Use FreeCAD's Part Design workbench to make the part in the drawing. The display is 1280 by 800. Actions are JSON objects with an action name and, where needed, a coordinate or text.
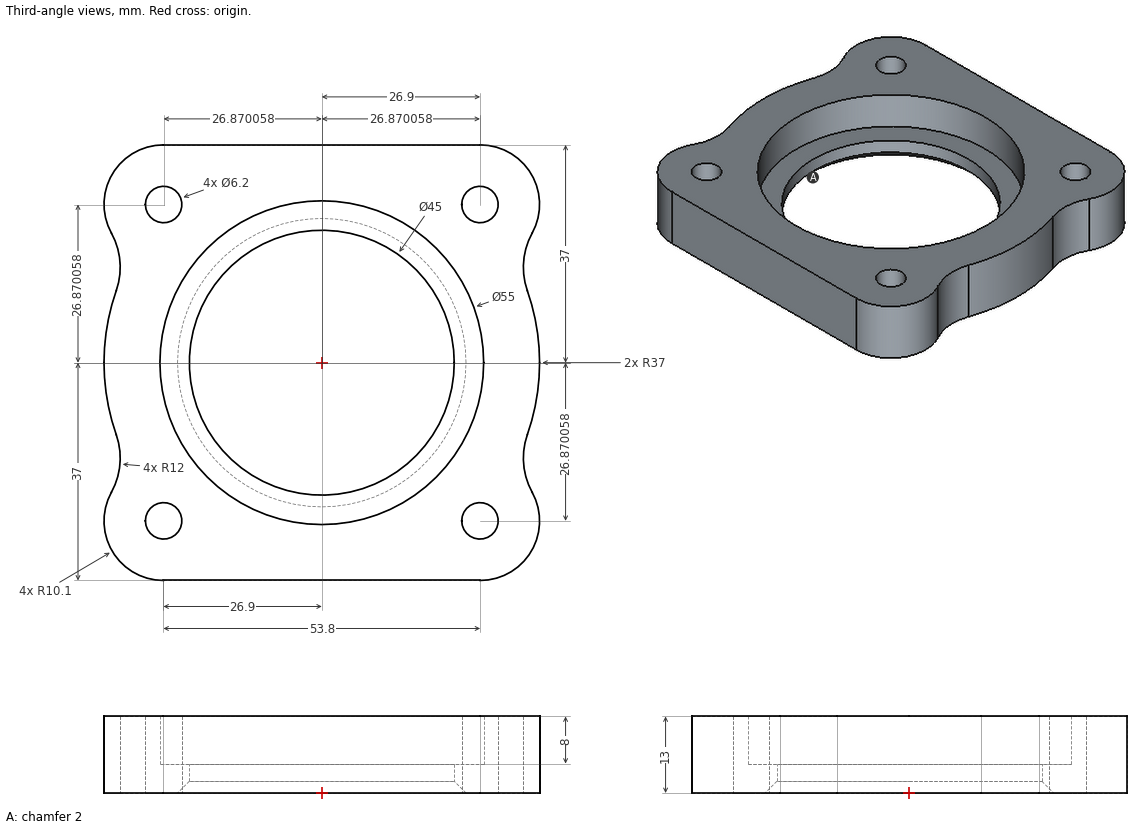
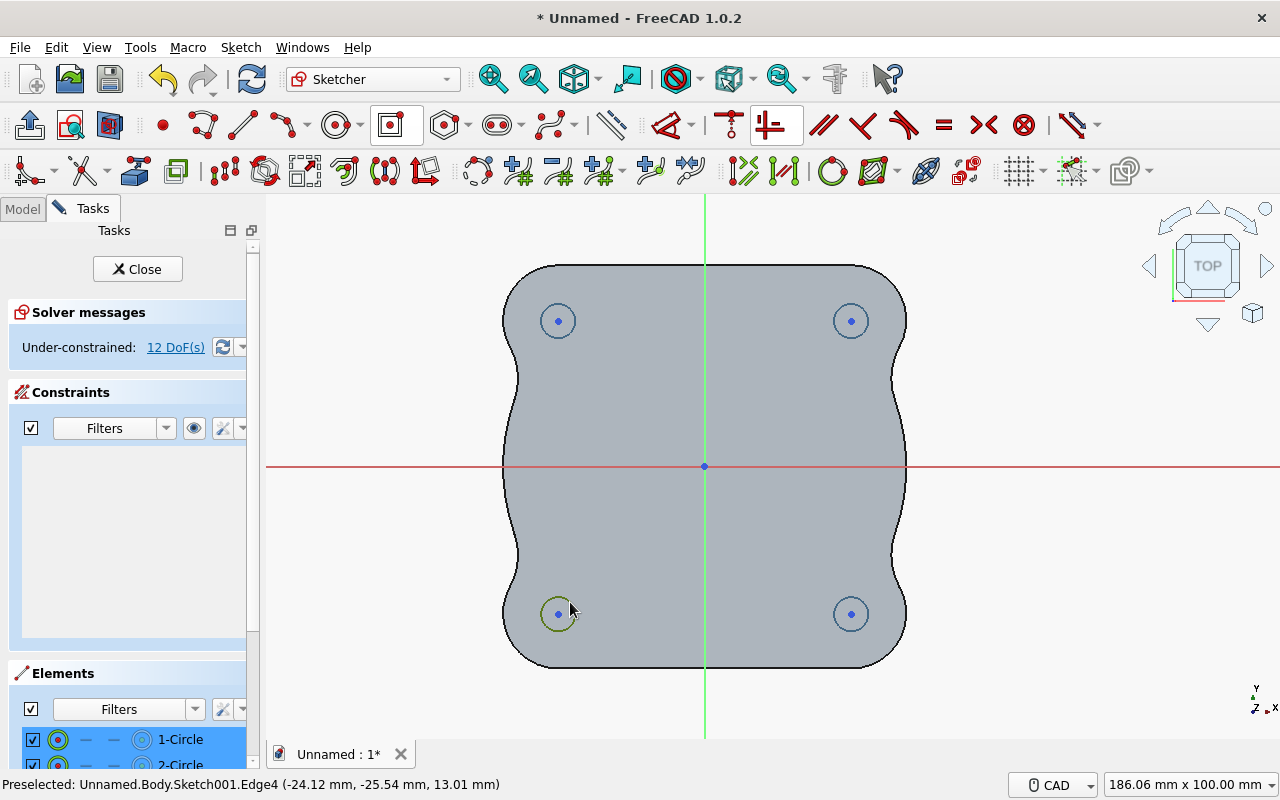
{"action": "key", "text": "e"}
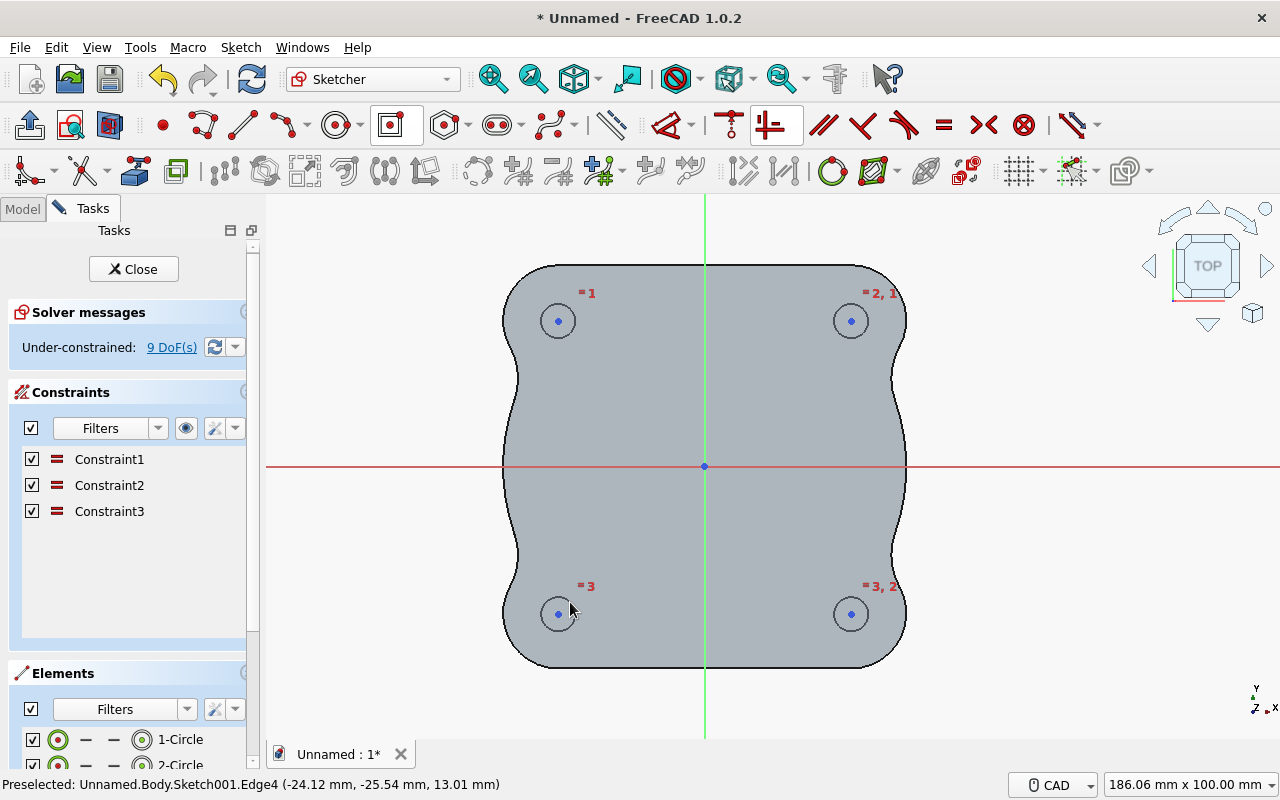
{"action": "left_click", "coordinate": [558, 321]}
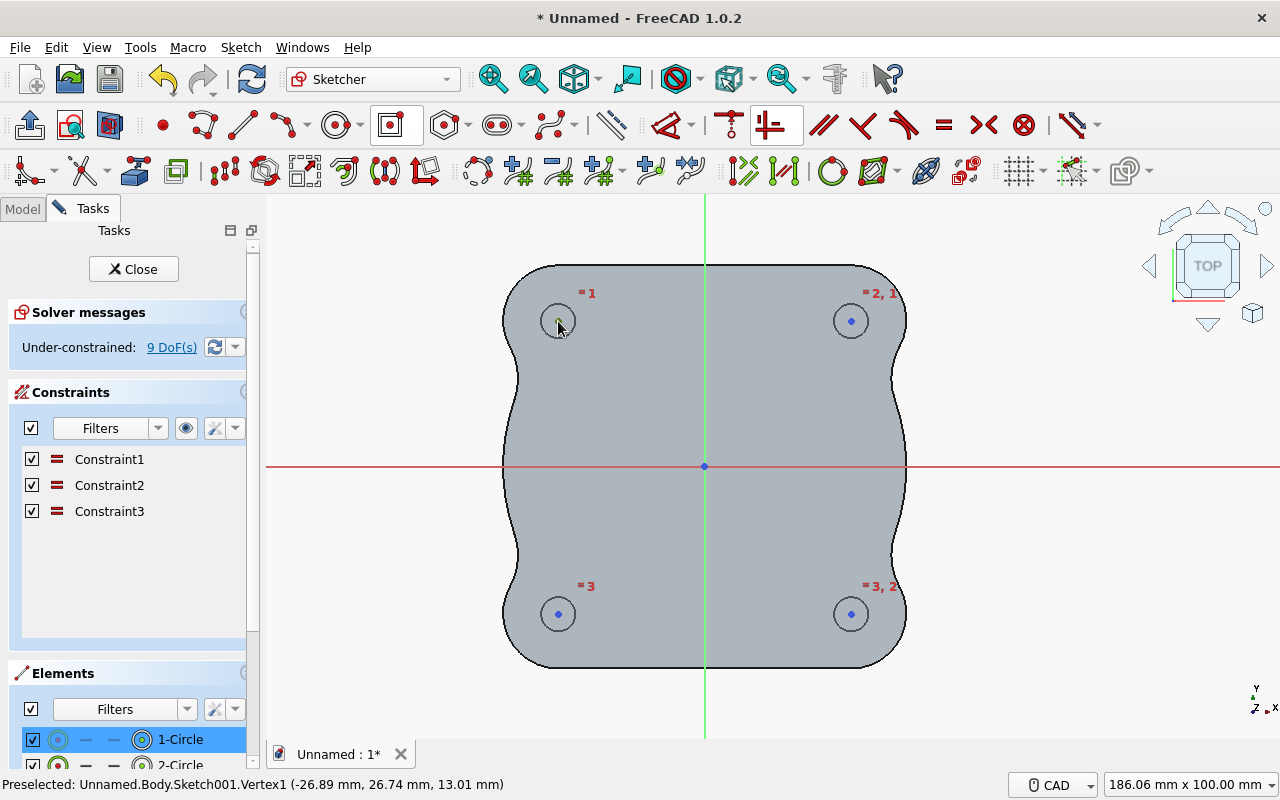
{"action": "left_click", "coordinate": [851, 321]}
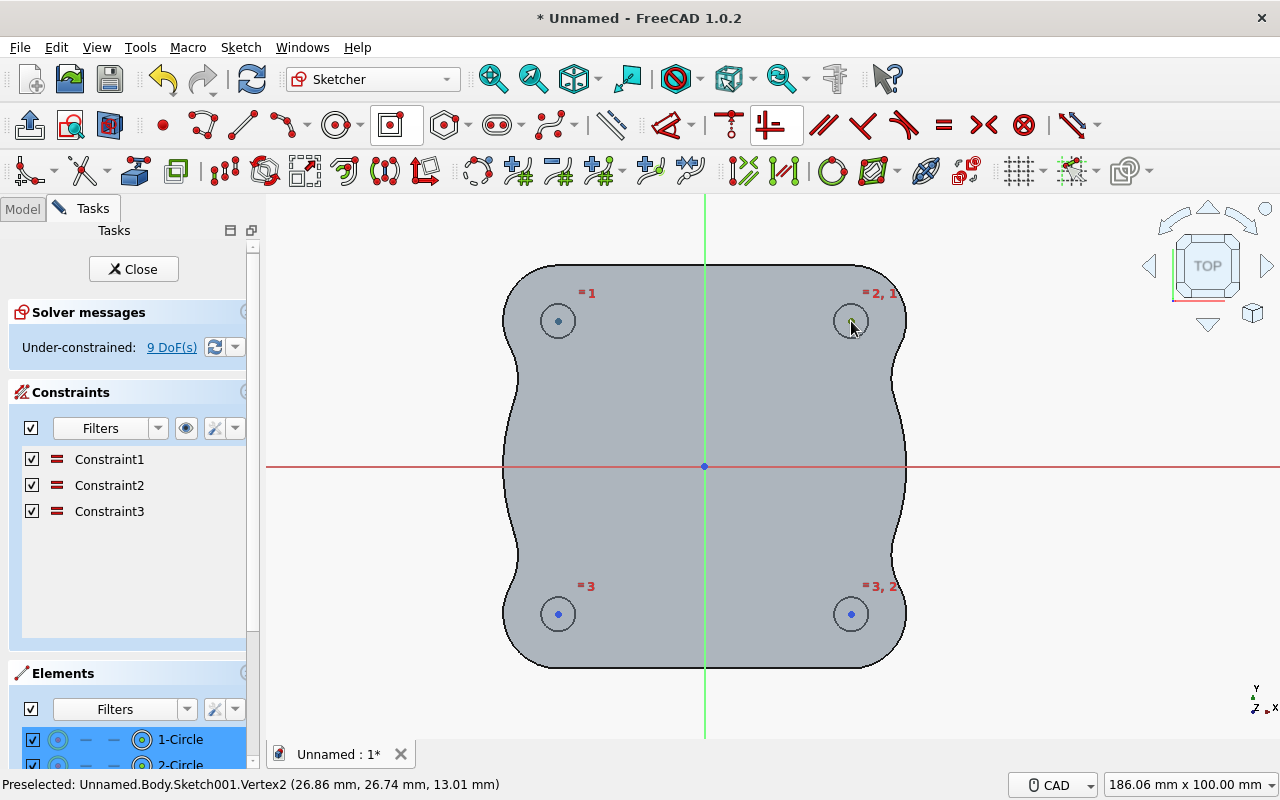
{"action": "key", "text": "h"}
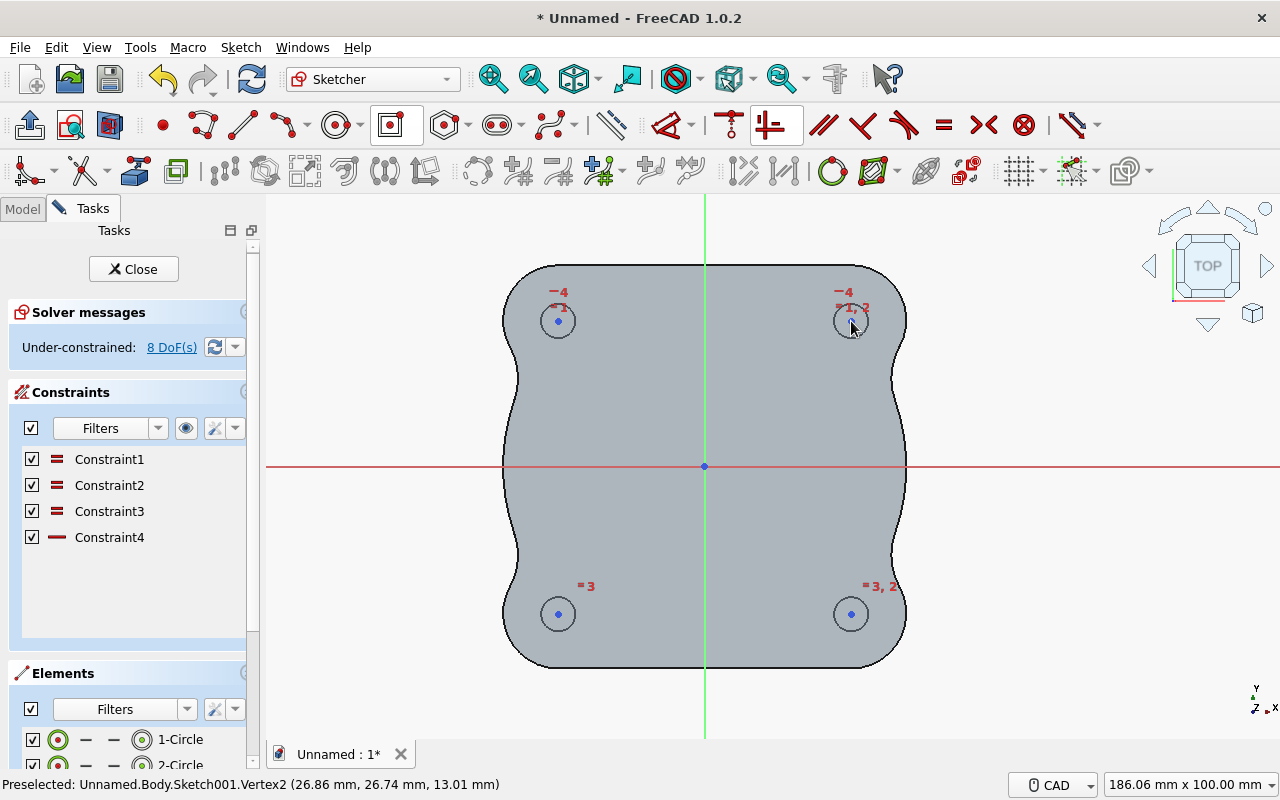
{"action": "left_click", "coordinate": [851, 321]}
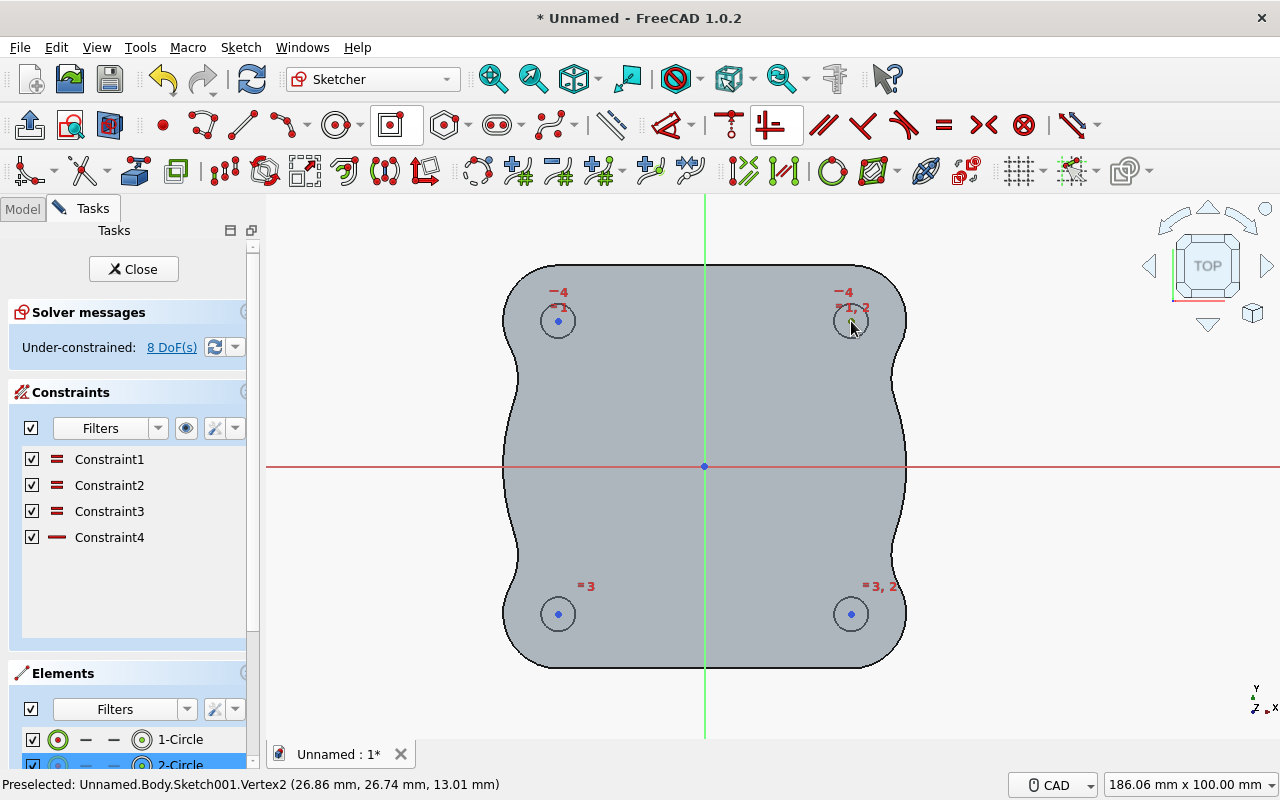
{"action": "left_click", "coordinate": [851, 614]}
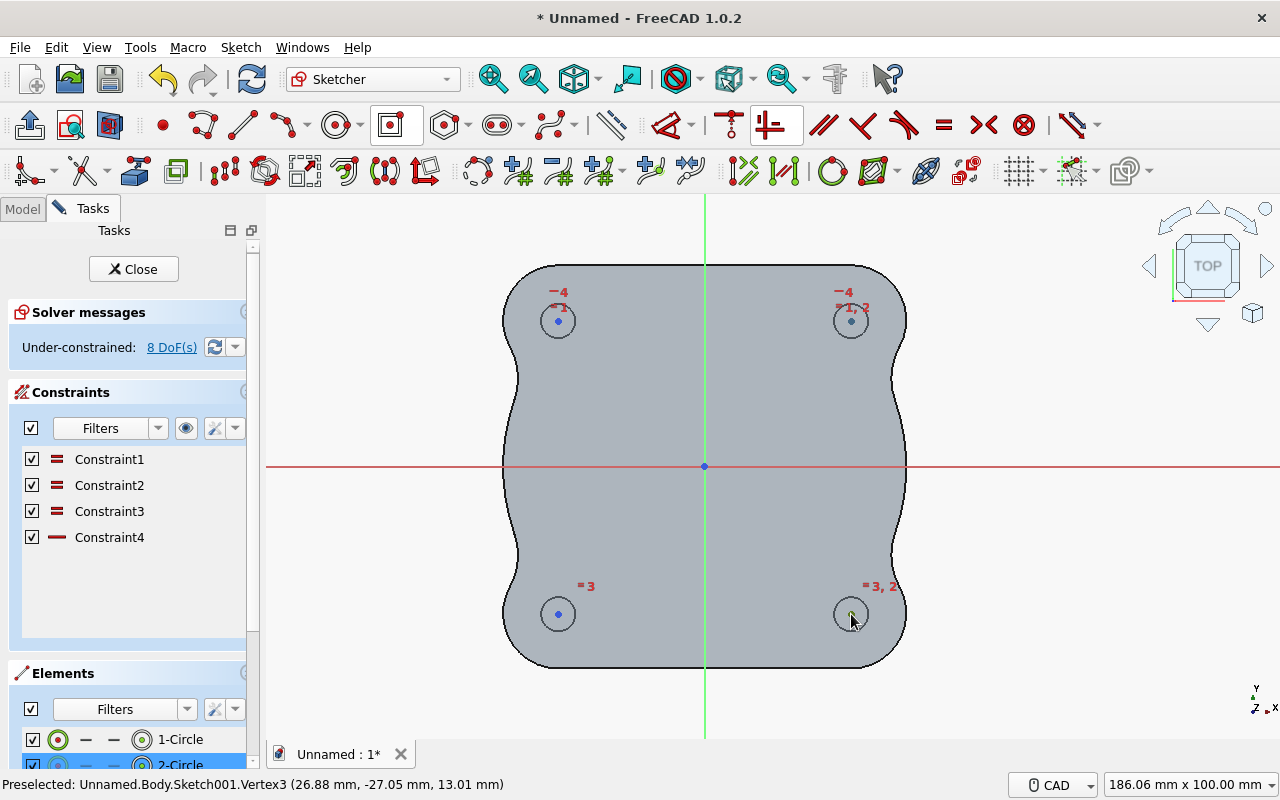
{"action": "key", "text": "v"}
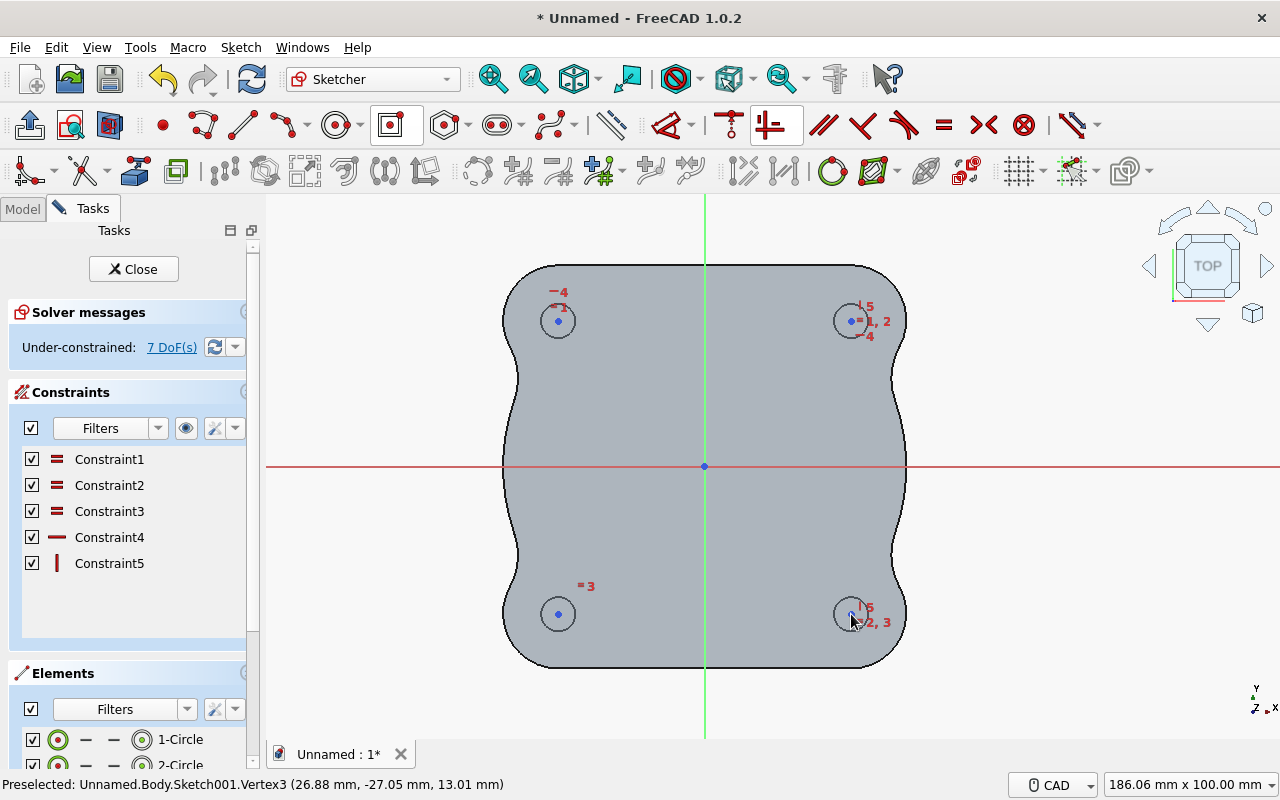
{"action": "left_click", "coordinate": [558, 321]}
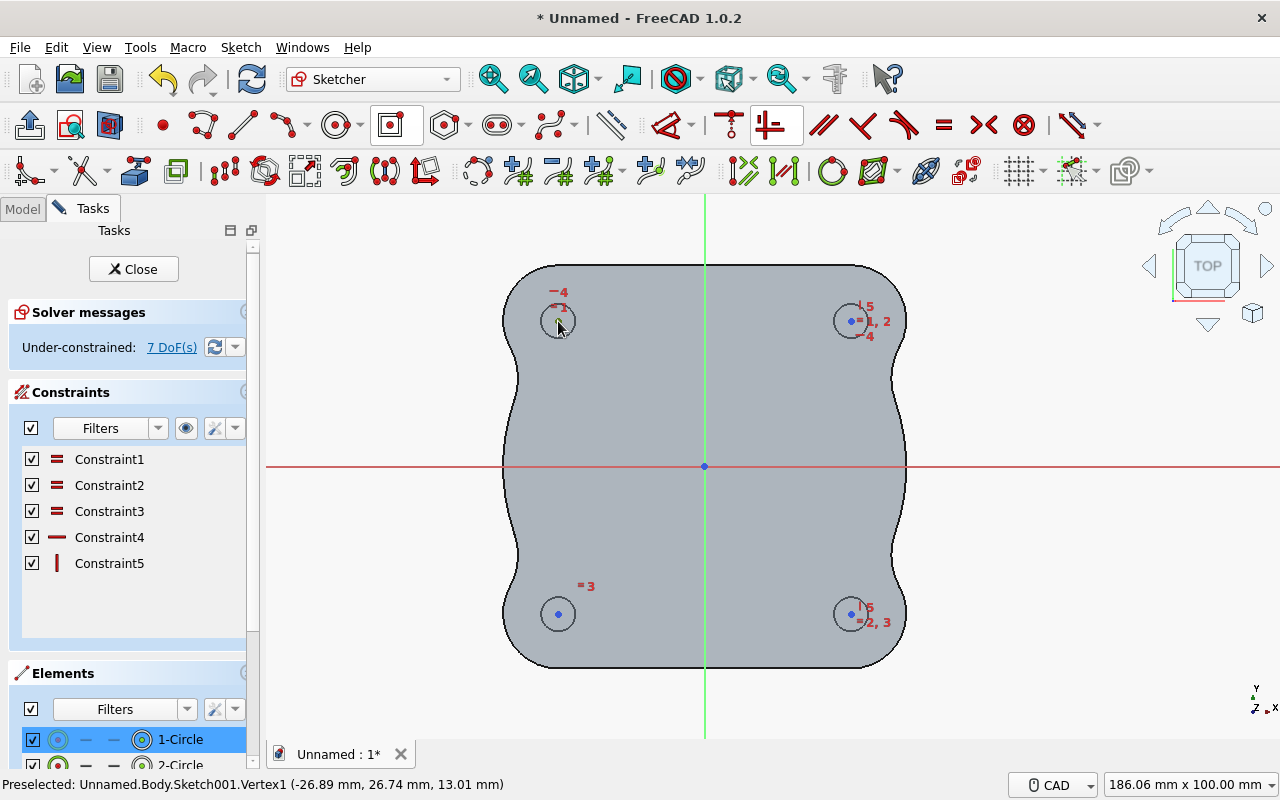
{"action": "left_click", "coordinate": [558, 614]}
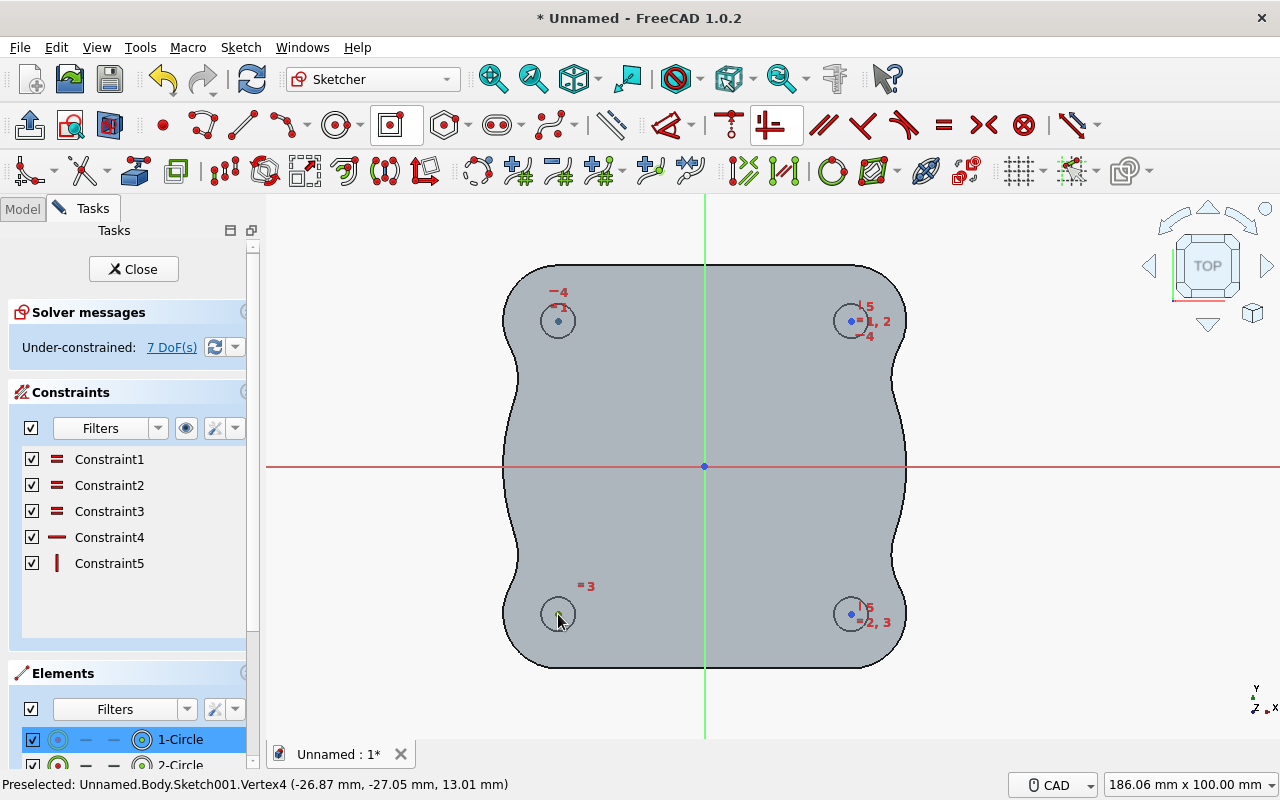
{"action": "key", "text": "v"}